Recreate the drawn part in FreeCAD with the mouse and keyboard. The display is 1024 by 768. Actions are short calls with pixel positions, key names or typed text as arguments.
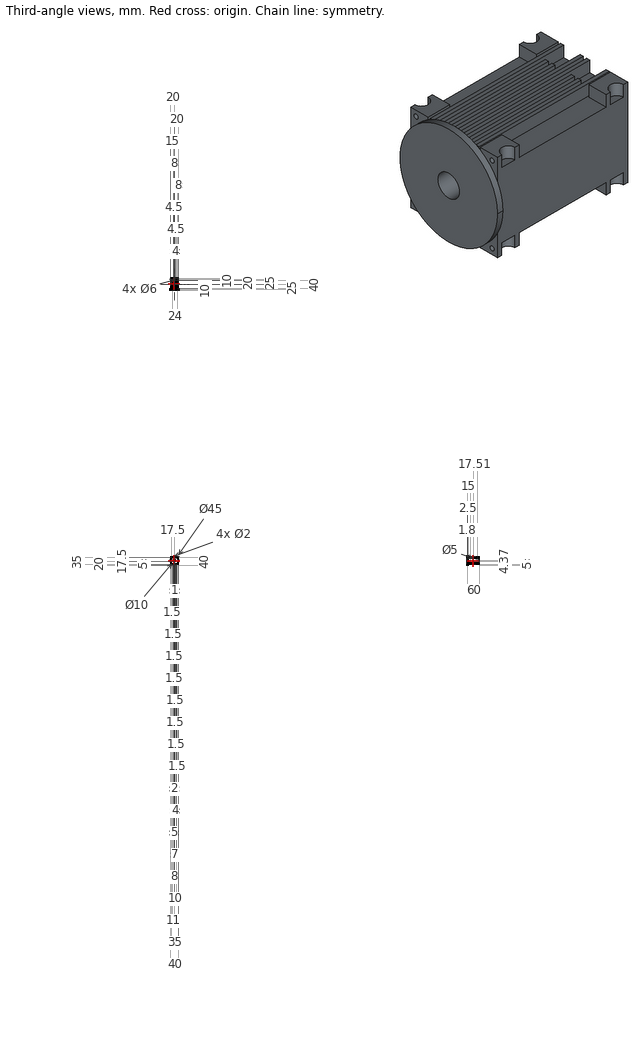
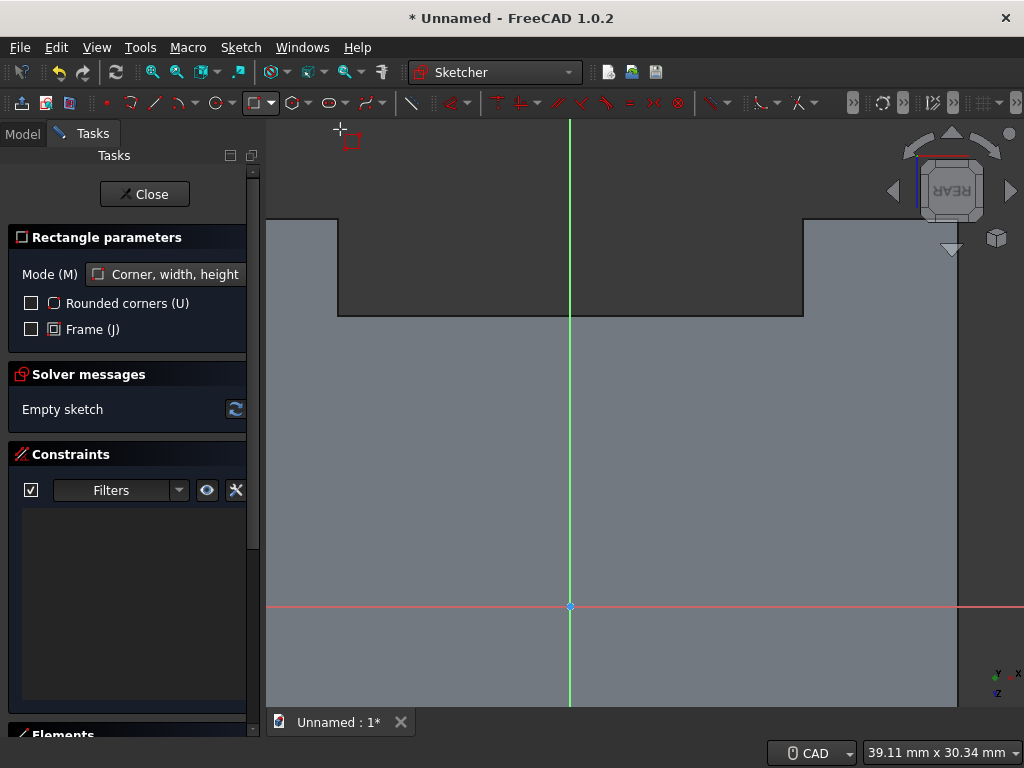
click(357, 219)
click(386, 316)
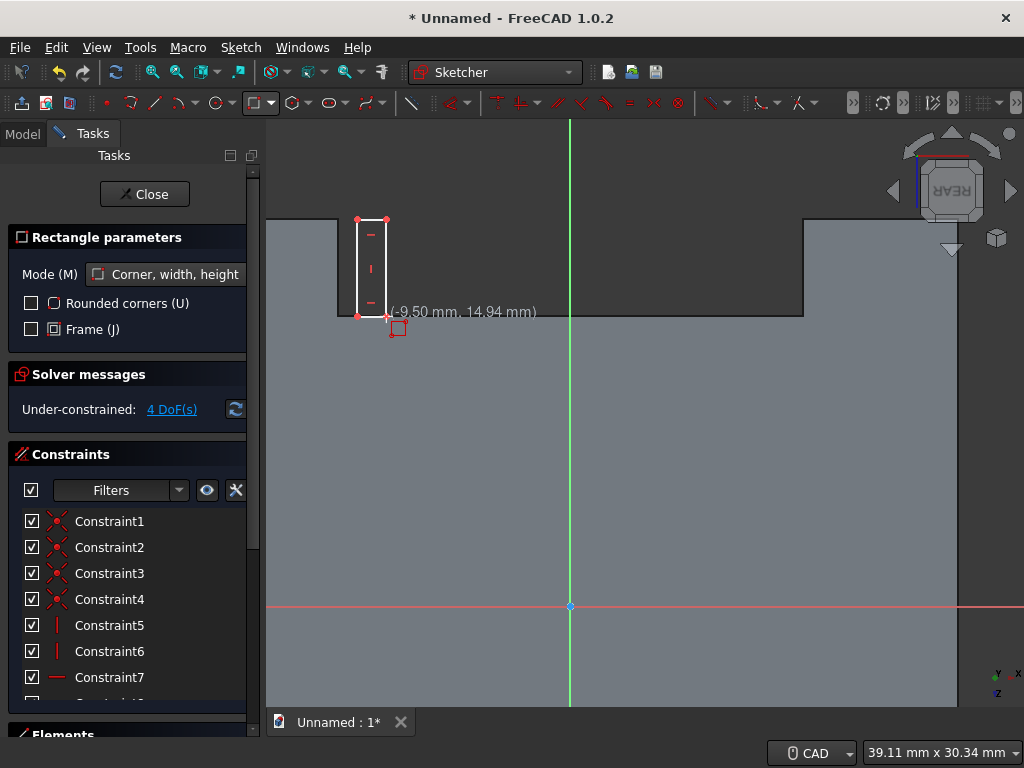
click(415, 219)
click(444, 316)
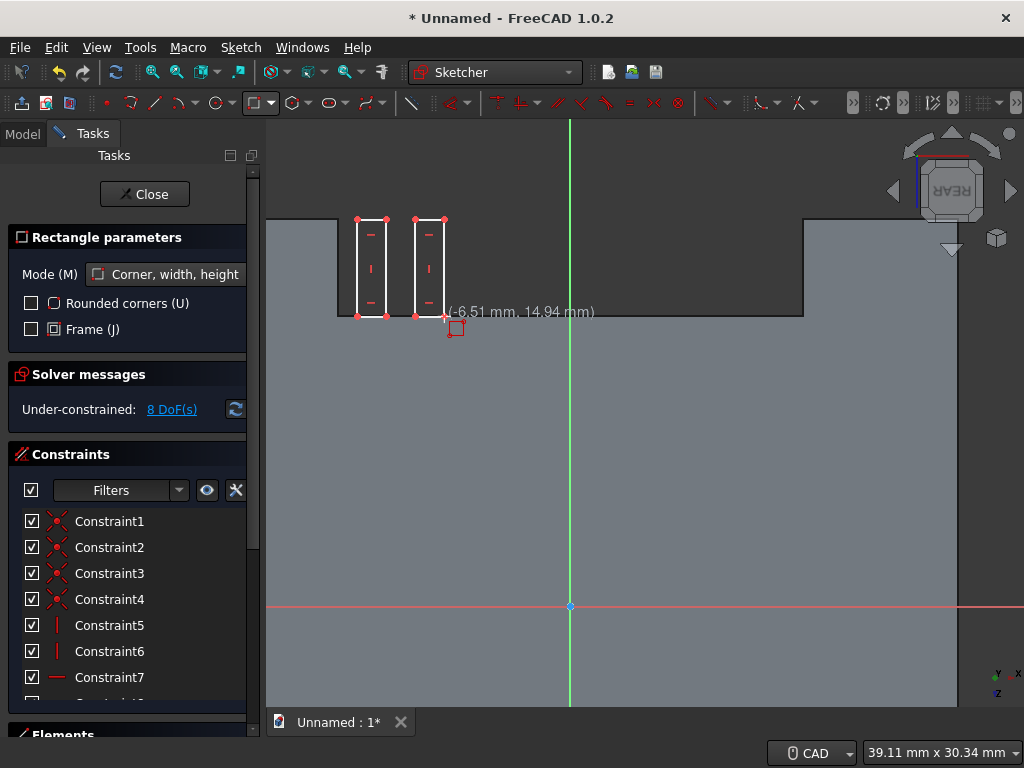
click(473, 219)
click(502, 316)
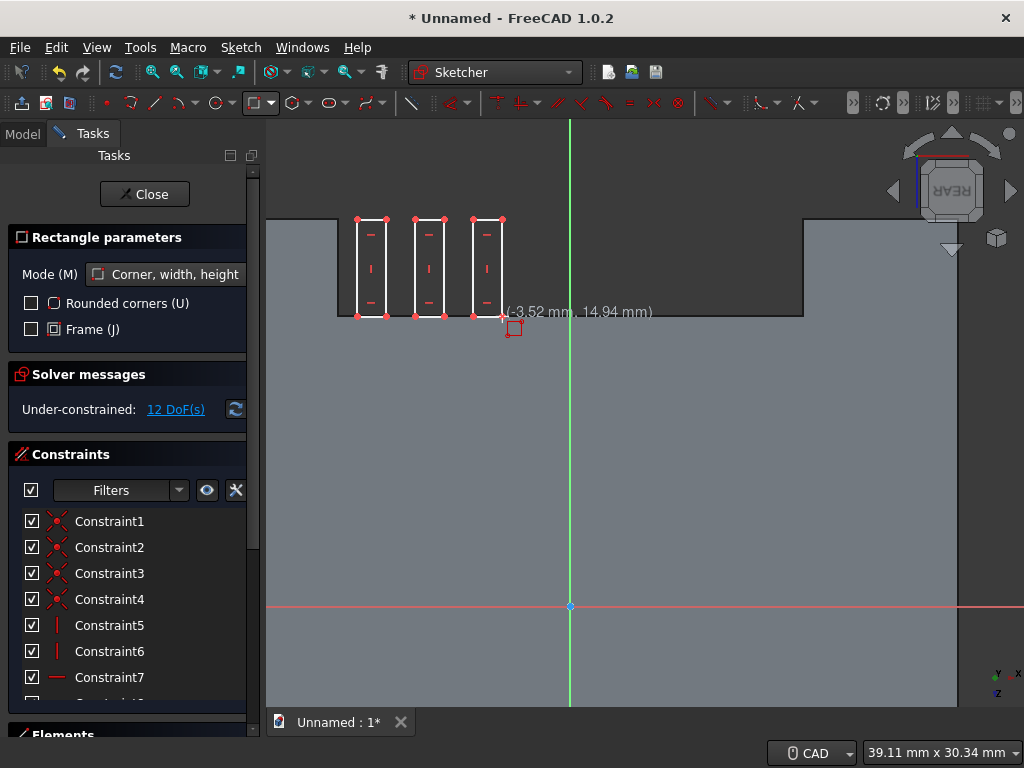
click(531, 219)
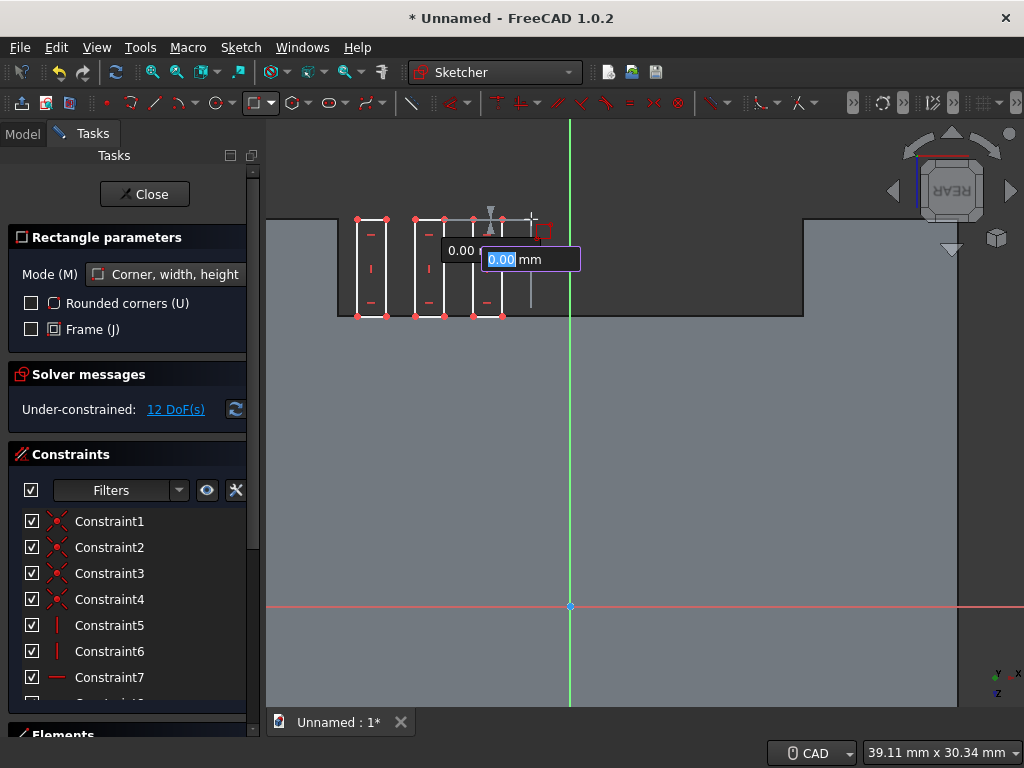
scroll(560, 316, up, 3)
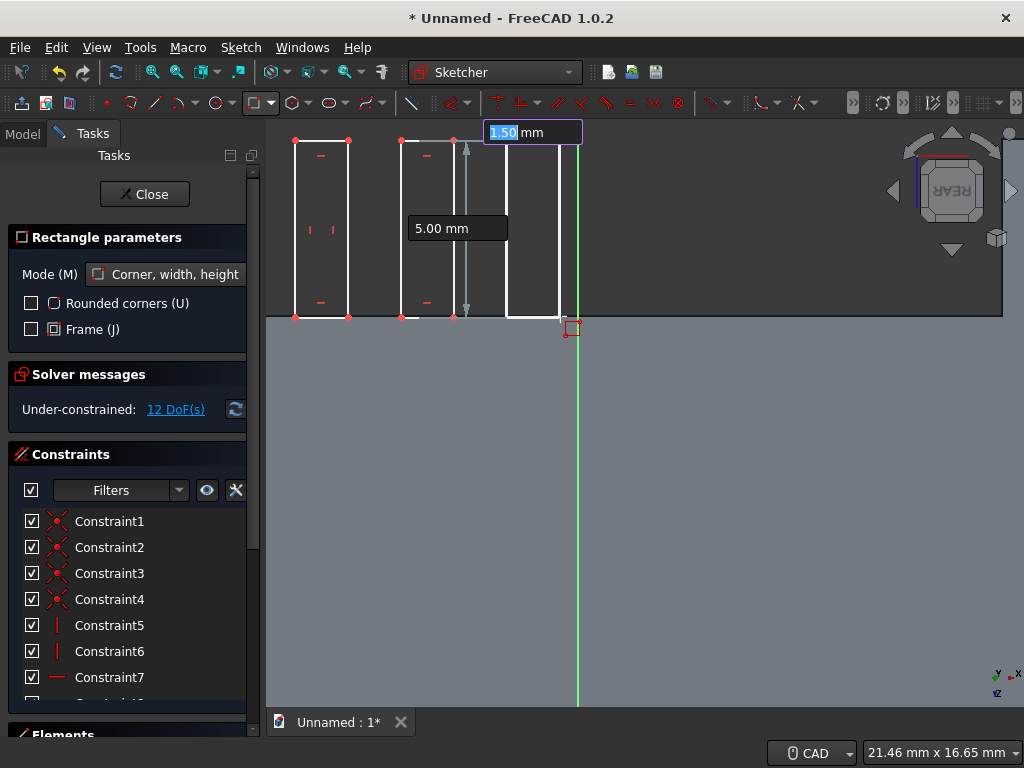
click(561, 316)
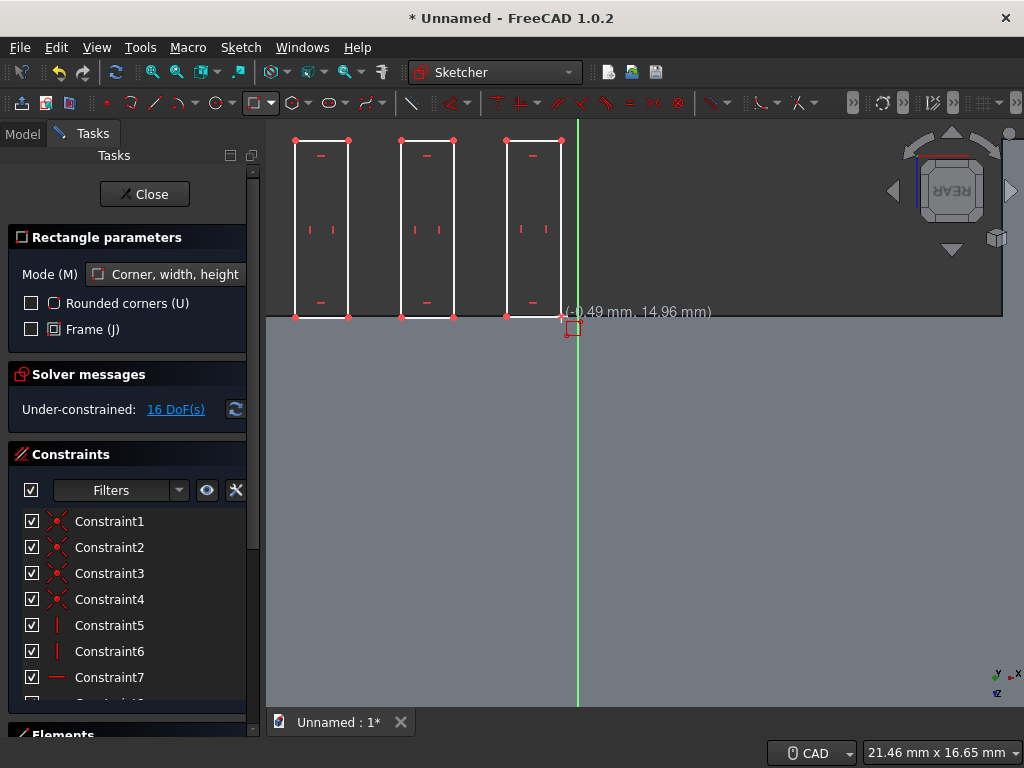
scroll(564, 317, down, 3)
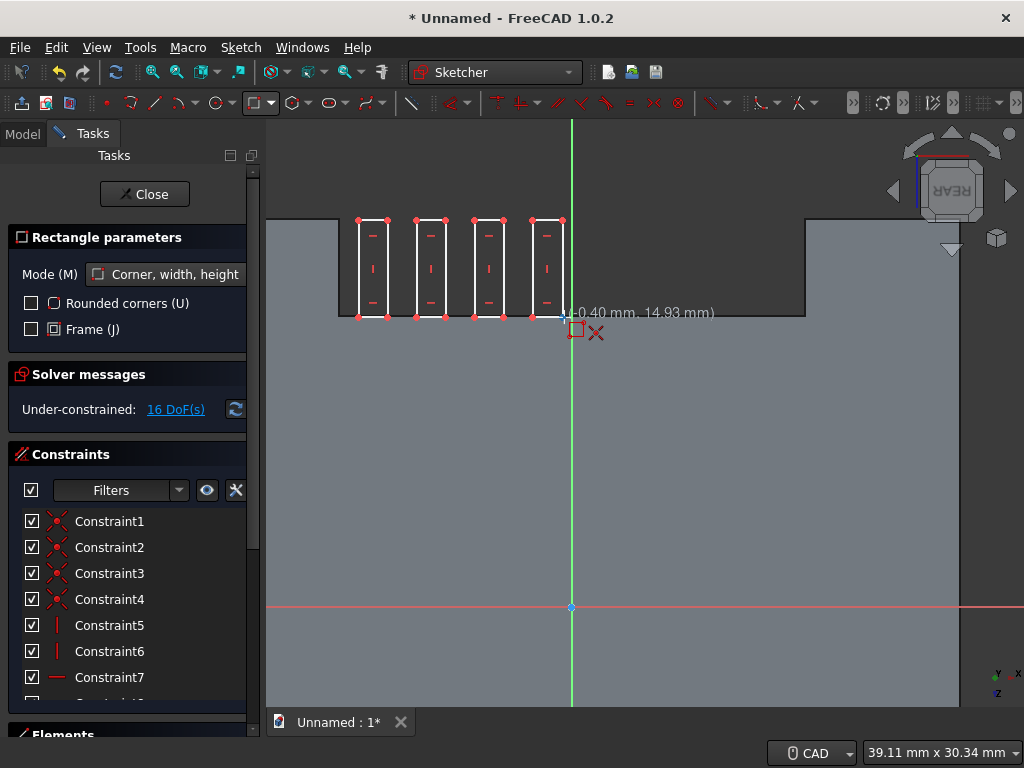
click(591, 219)
click(620, 316)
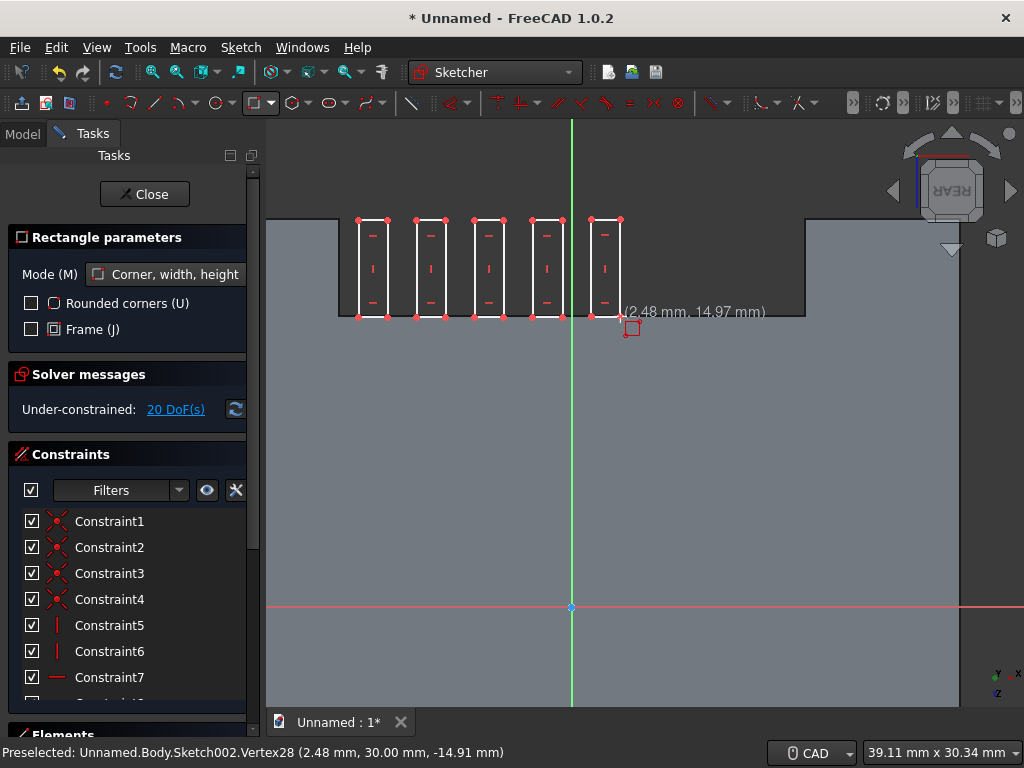
click(649, 219)
click(679, 316)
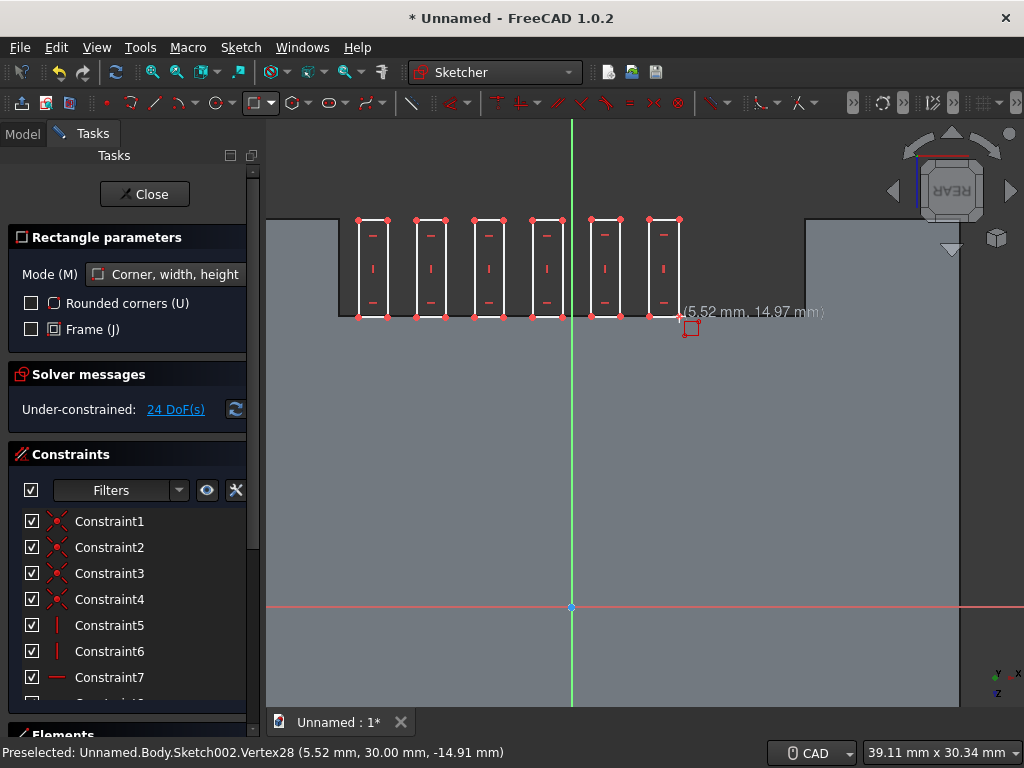
click(708, 219)
click(737, 316)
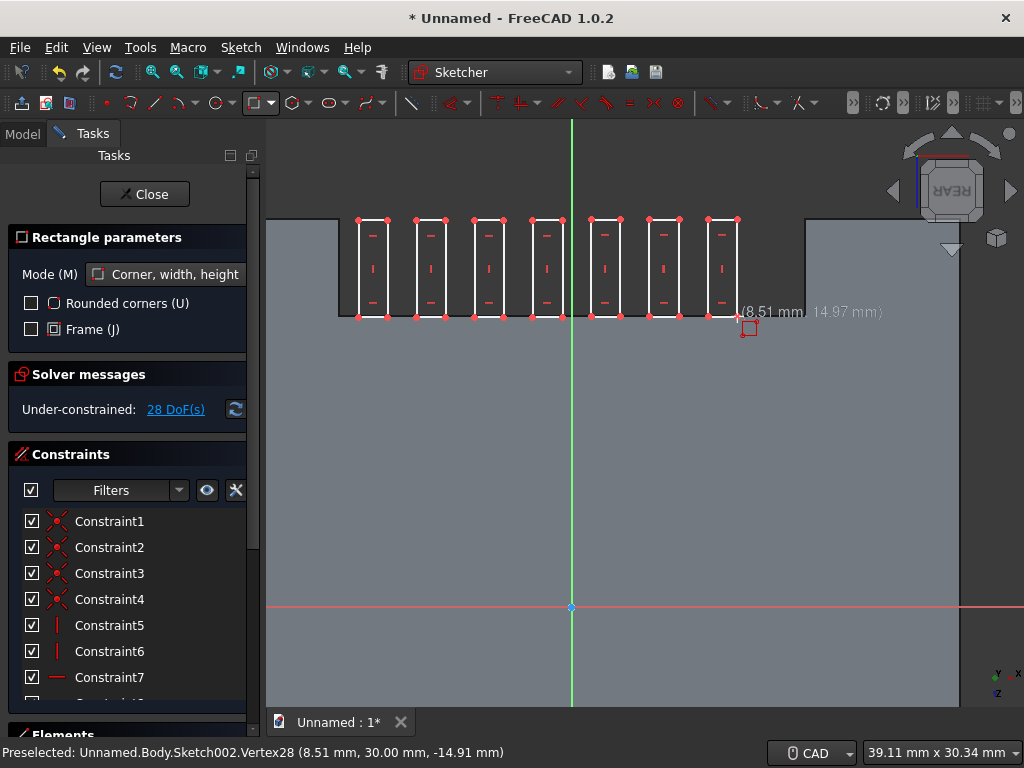
click(766, 219)
click(795, 316)
key(Escape)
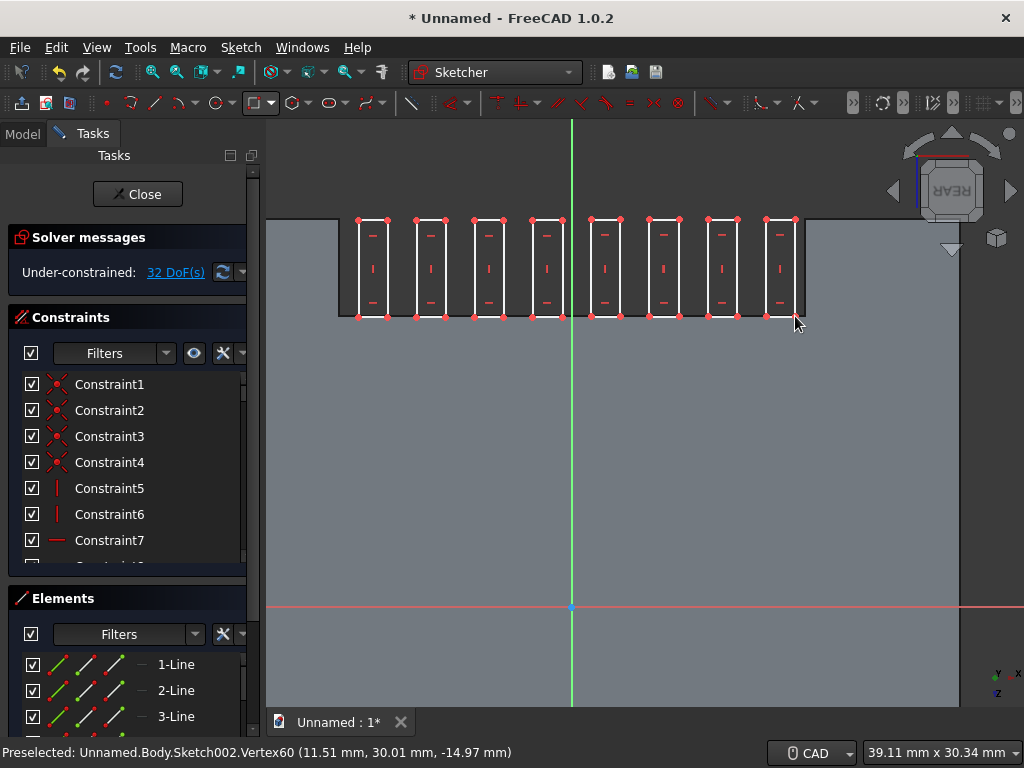
click(450, 104)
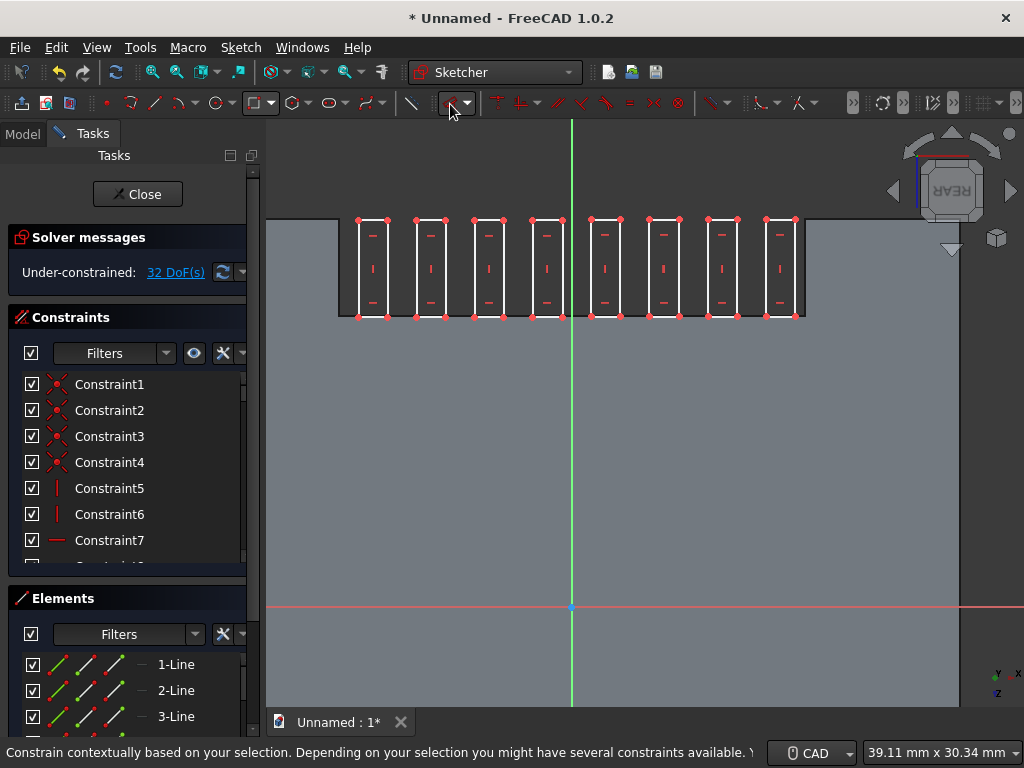
click(359, 250)
click(325, 269)